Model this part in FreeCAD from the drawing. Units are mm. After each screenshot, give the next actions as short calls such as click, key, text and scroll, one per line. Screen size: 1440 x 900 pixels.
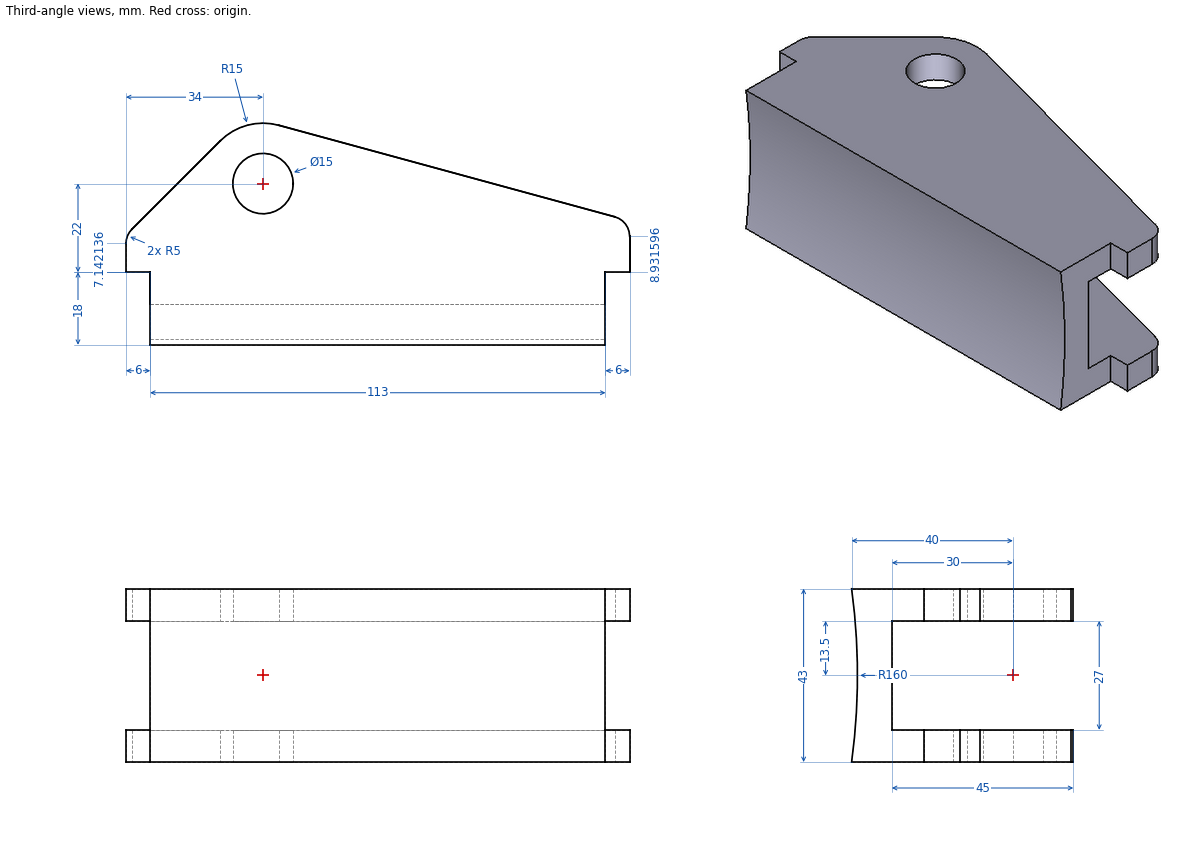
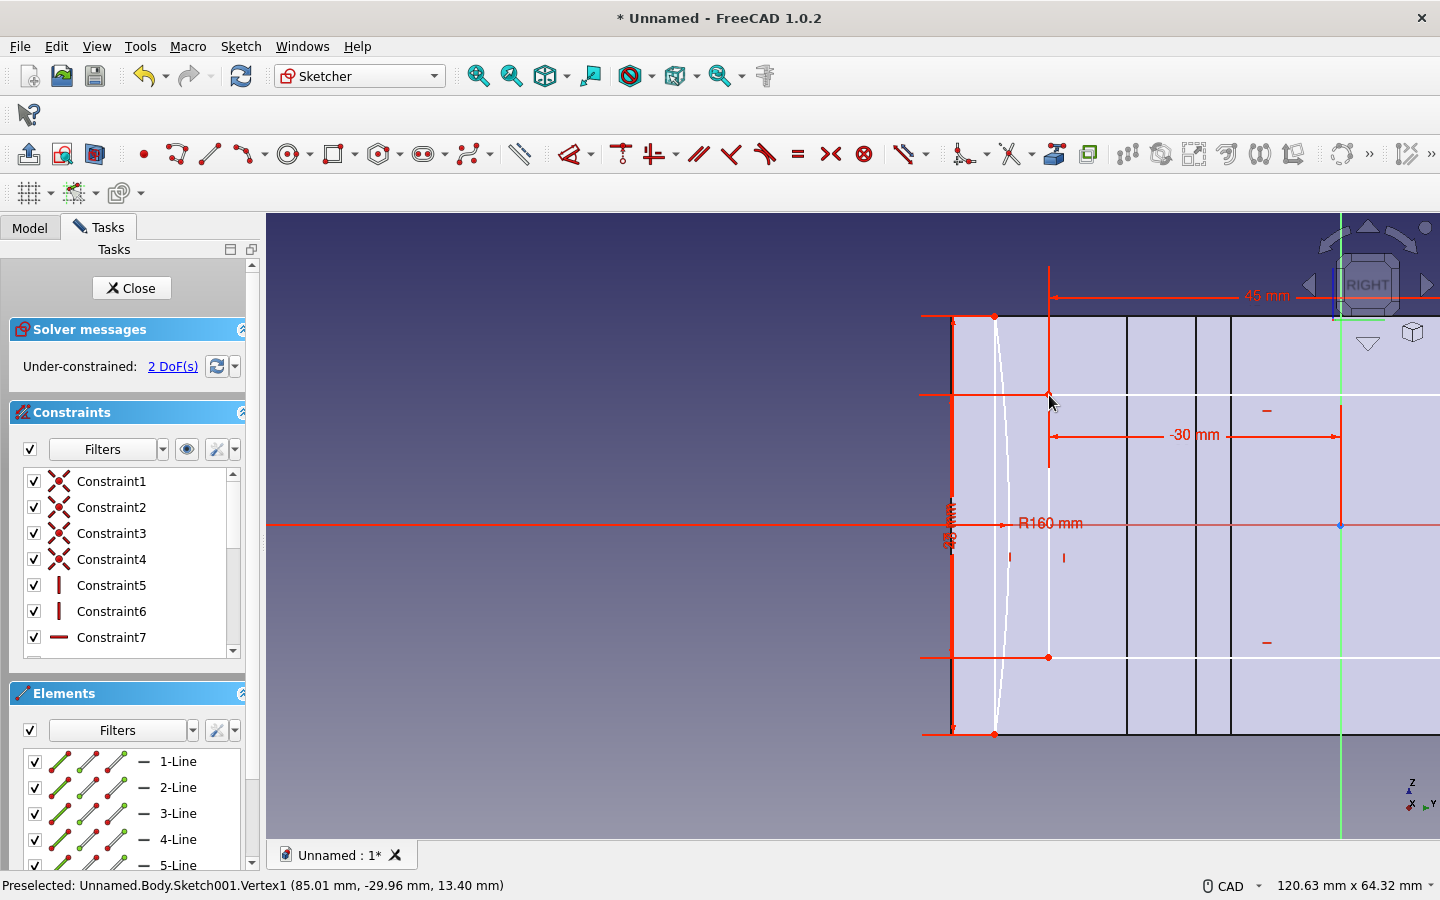
click(995, 316)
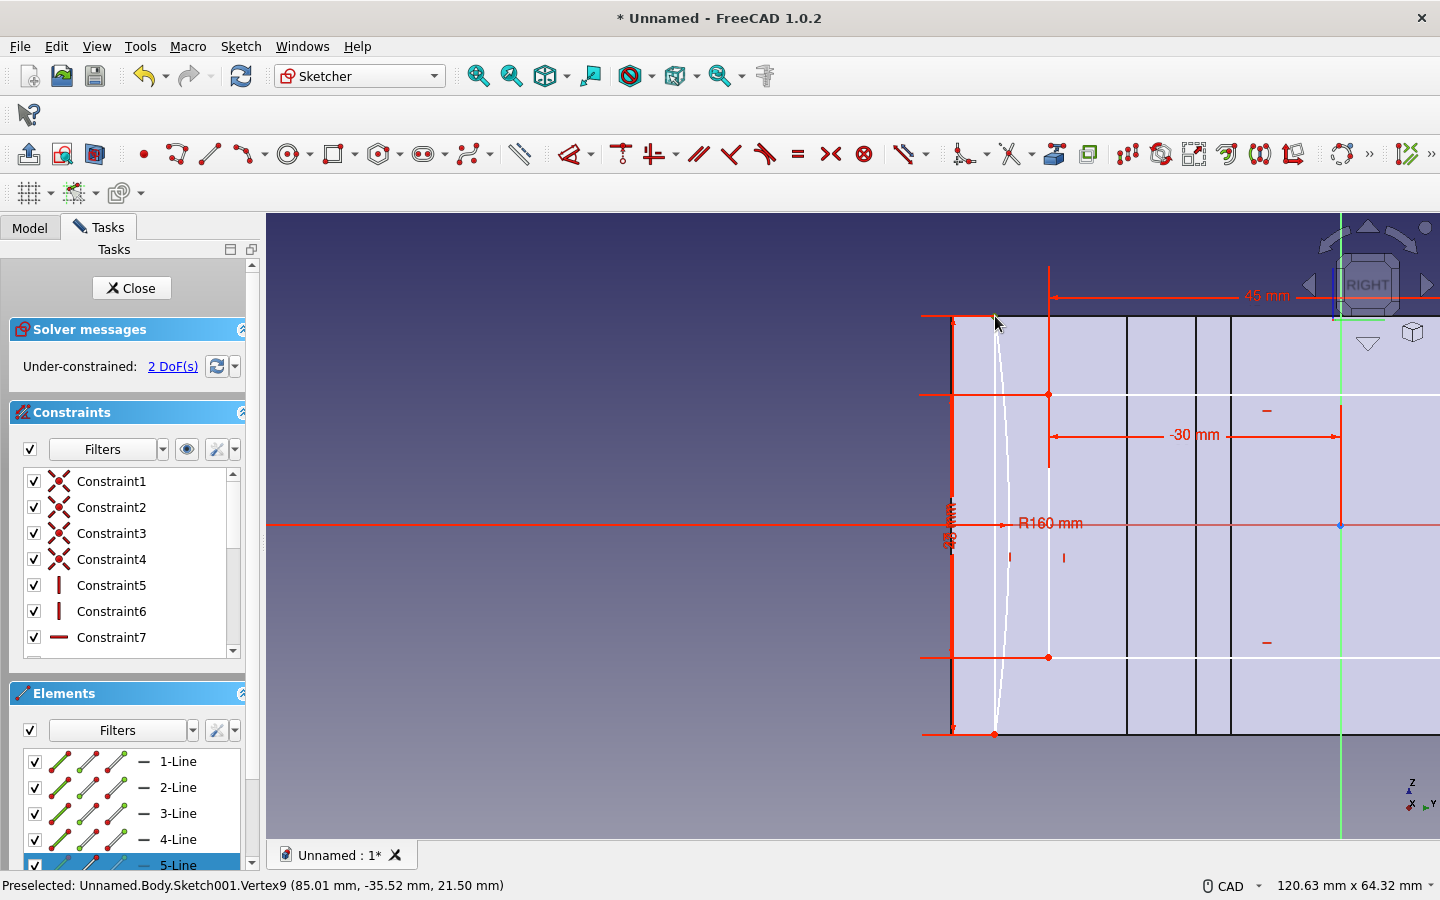
key(l)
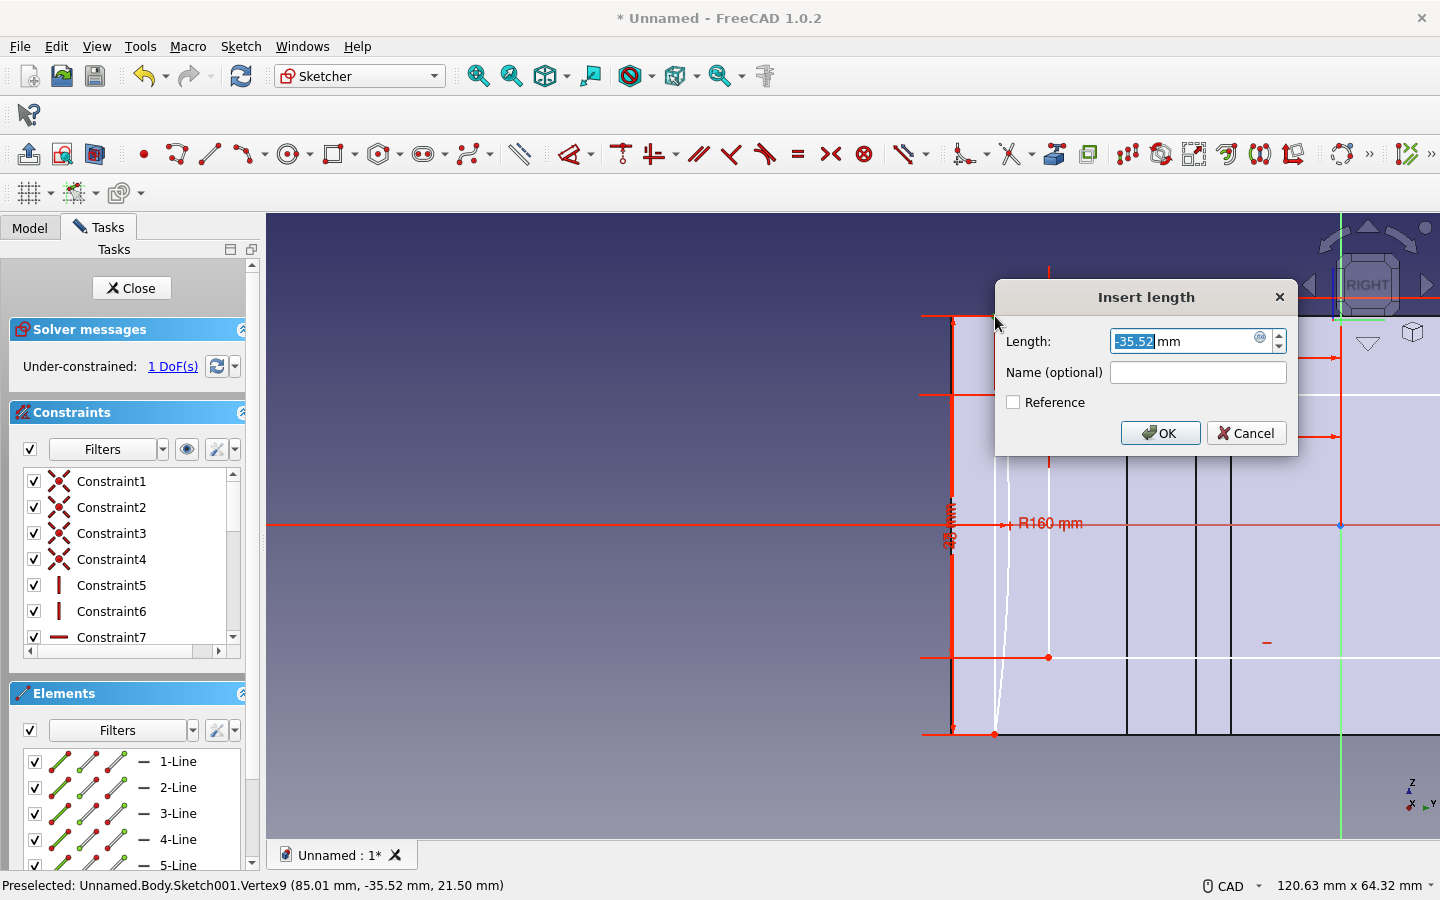
text(-40)
key(Return)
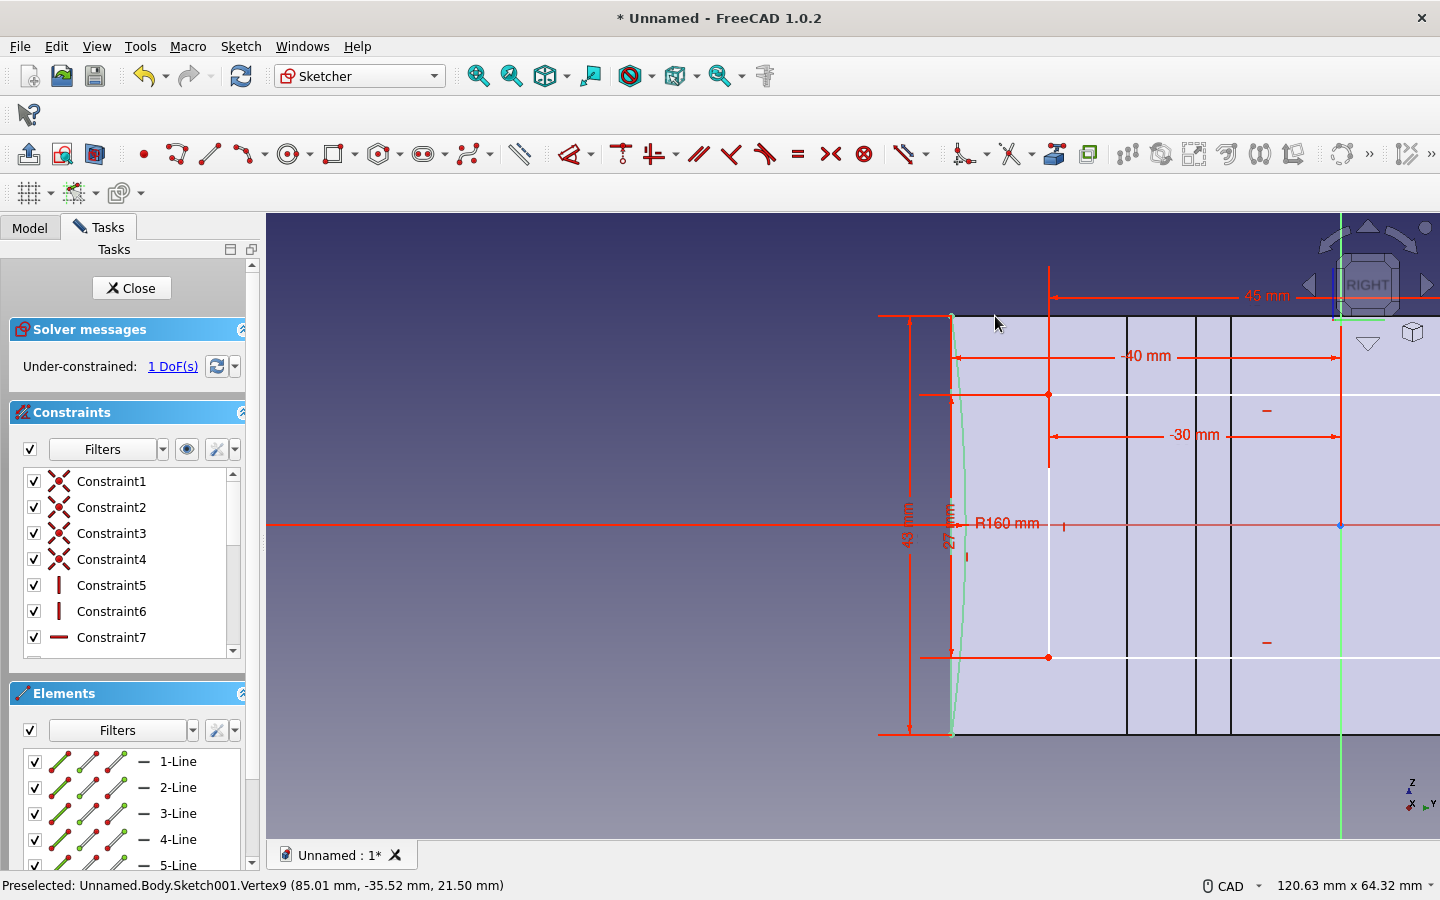
click(1049, 395)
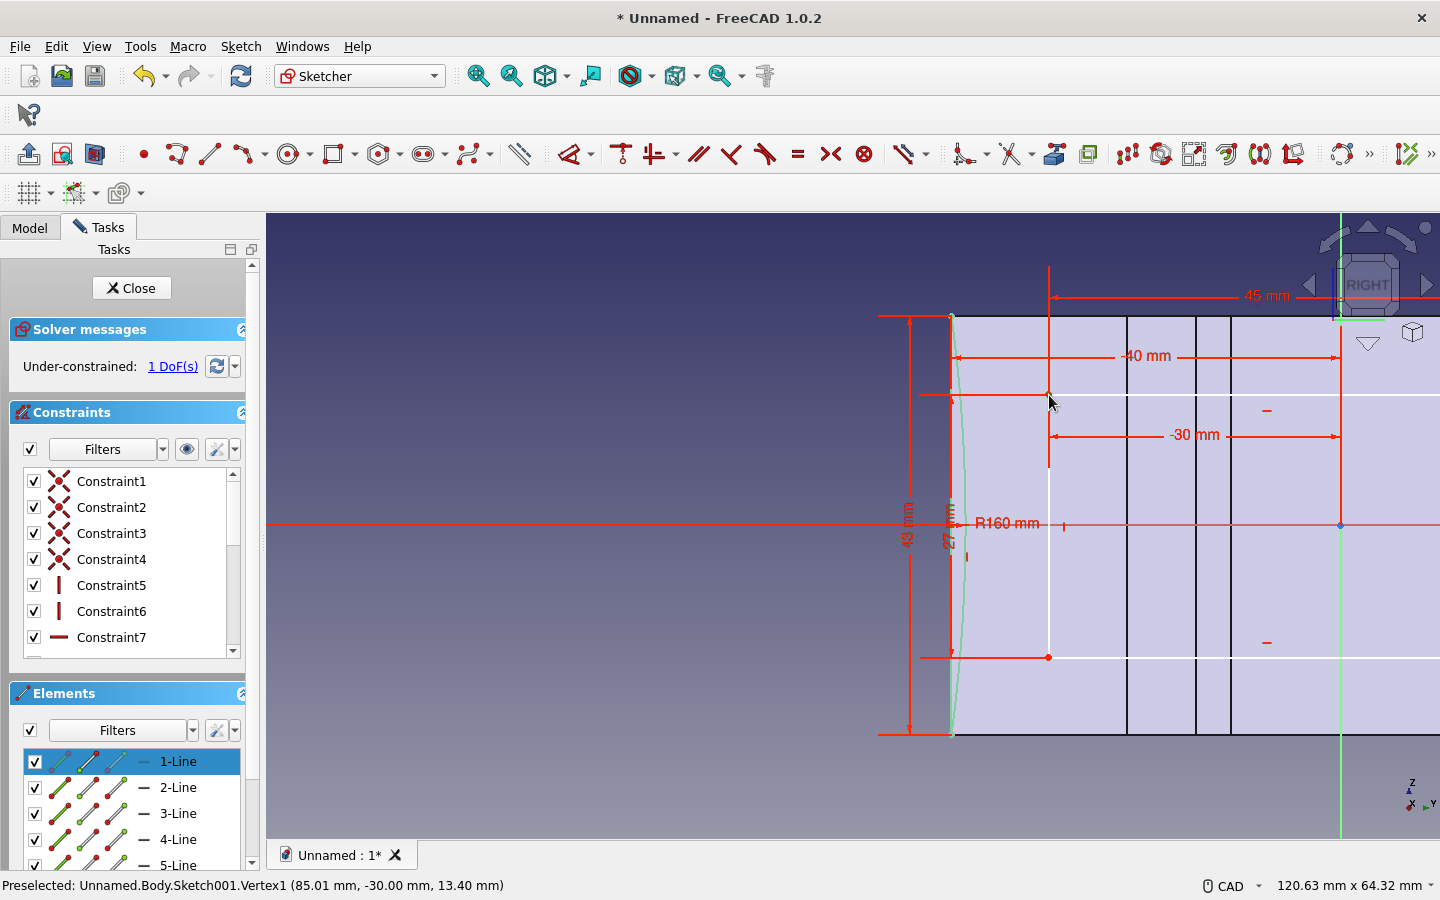
key(i)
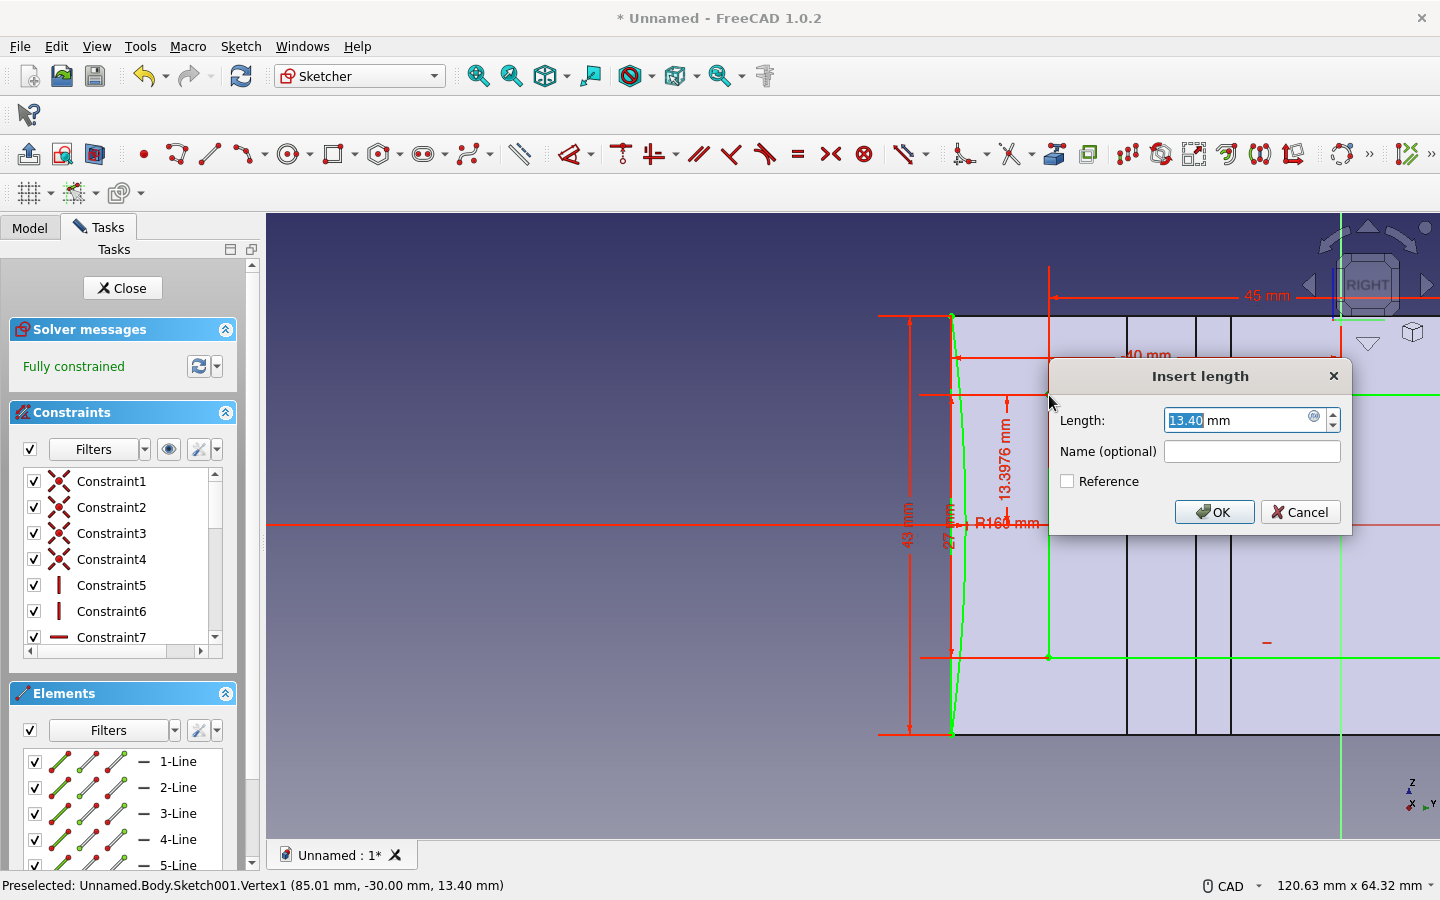
text(13.5)
key(Return)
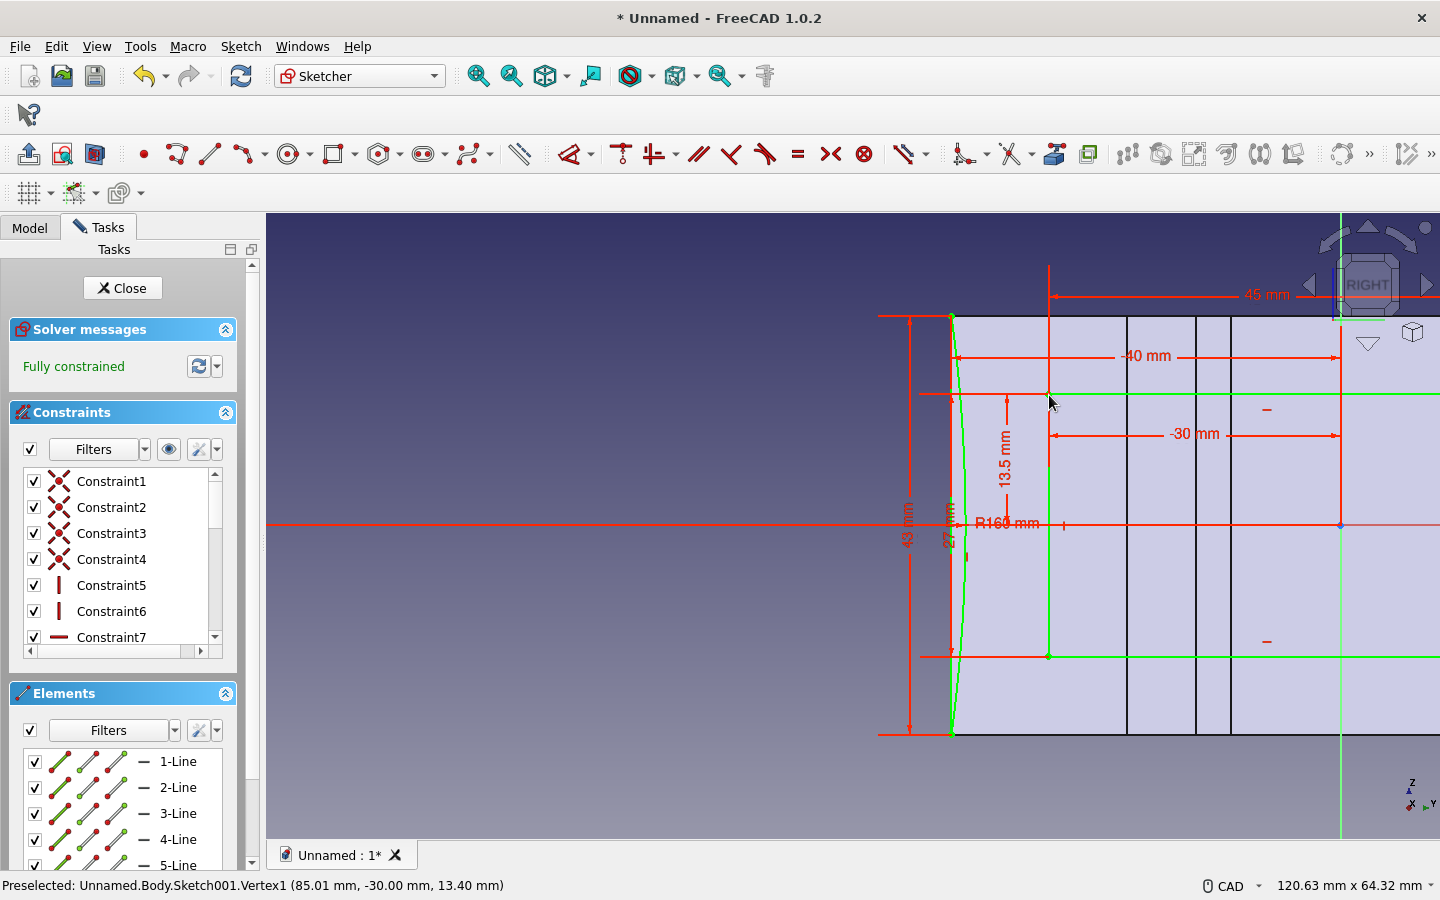
click(123, 288)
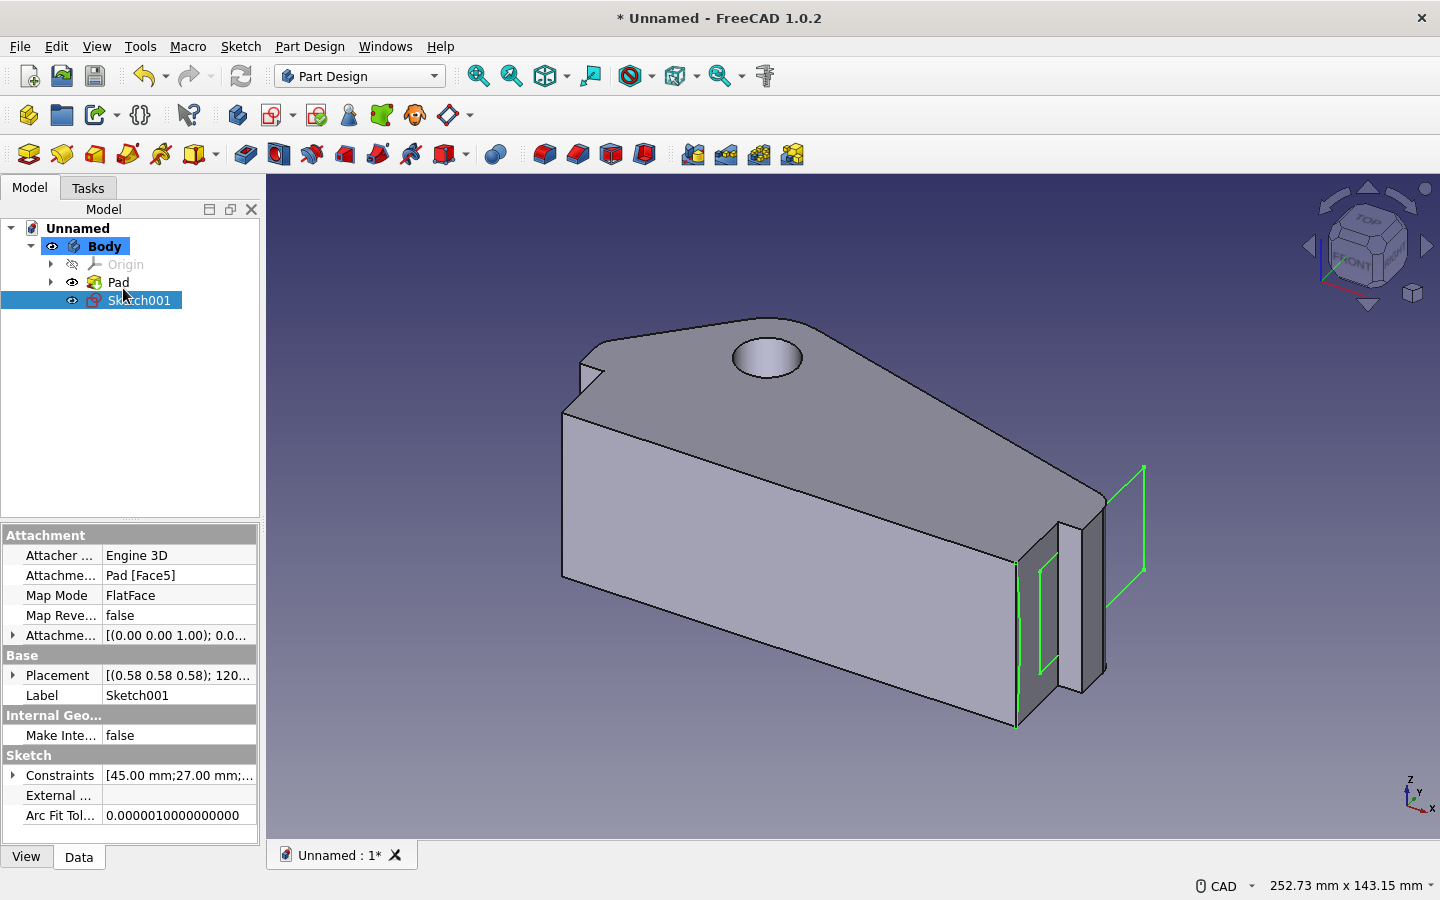
click(246, 154)